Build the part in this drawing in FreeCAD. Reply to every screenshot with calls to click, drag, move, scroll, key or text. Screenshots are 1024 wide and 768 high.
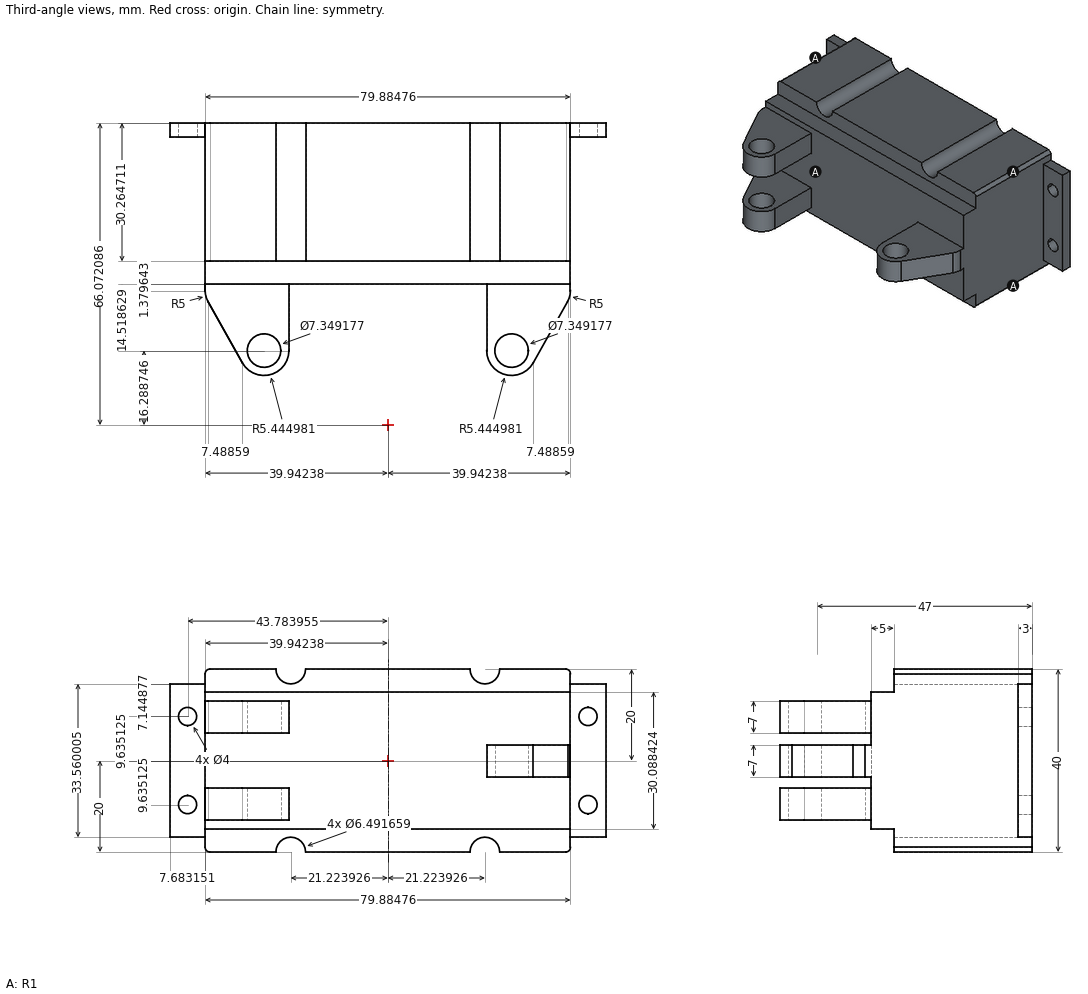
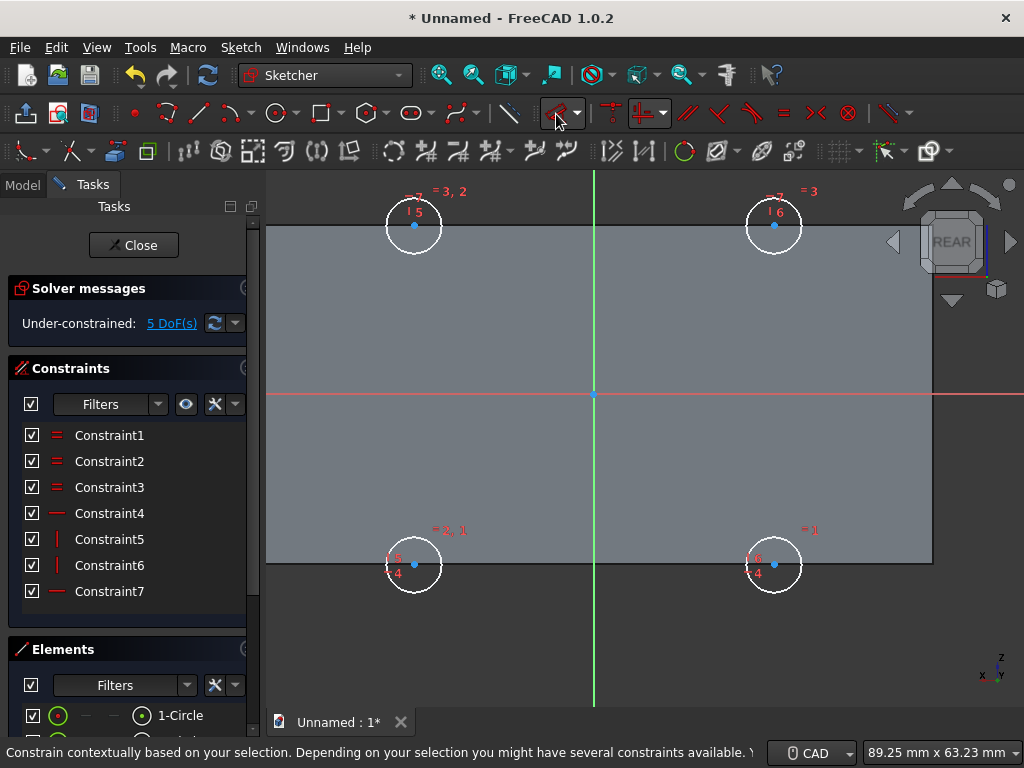
click(793, 545)
click(815, 522)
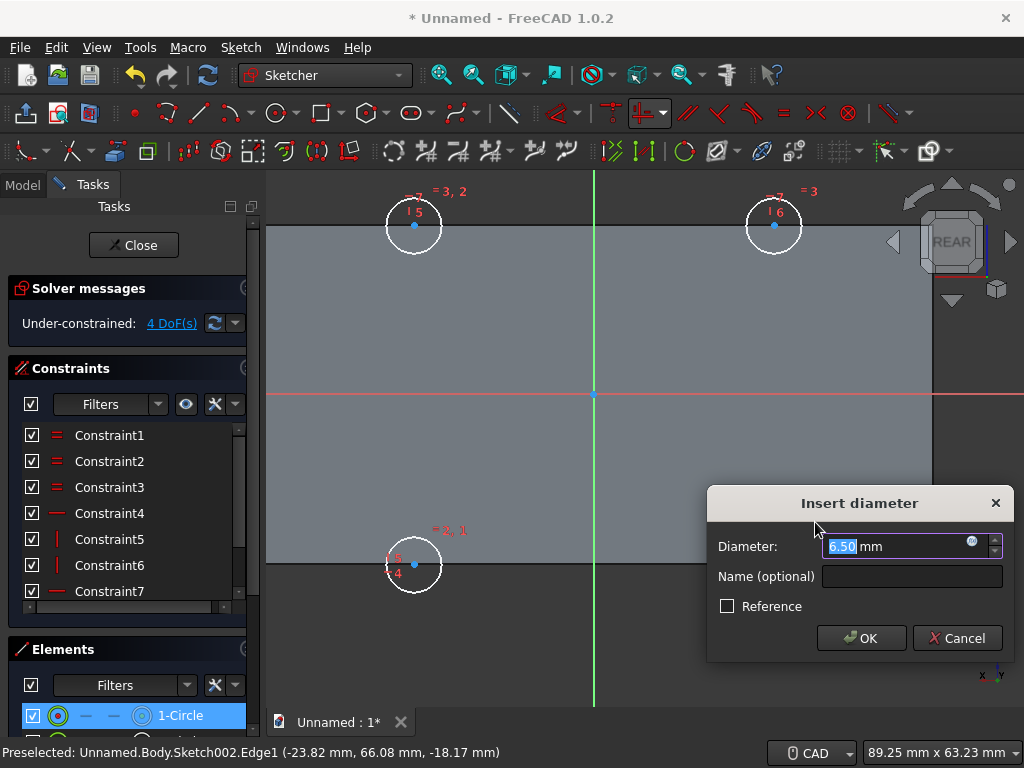
text(6.491659)
key(Return)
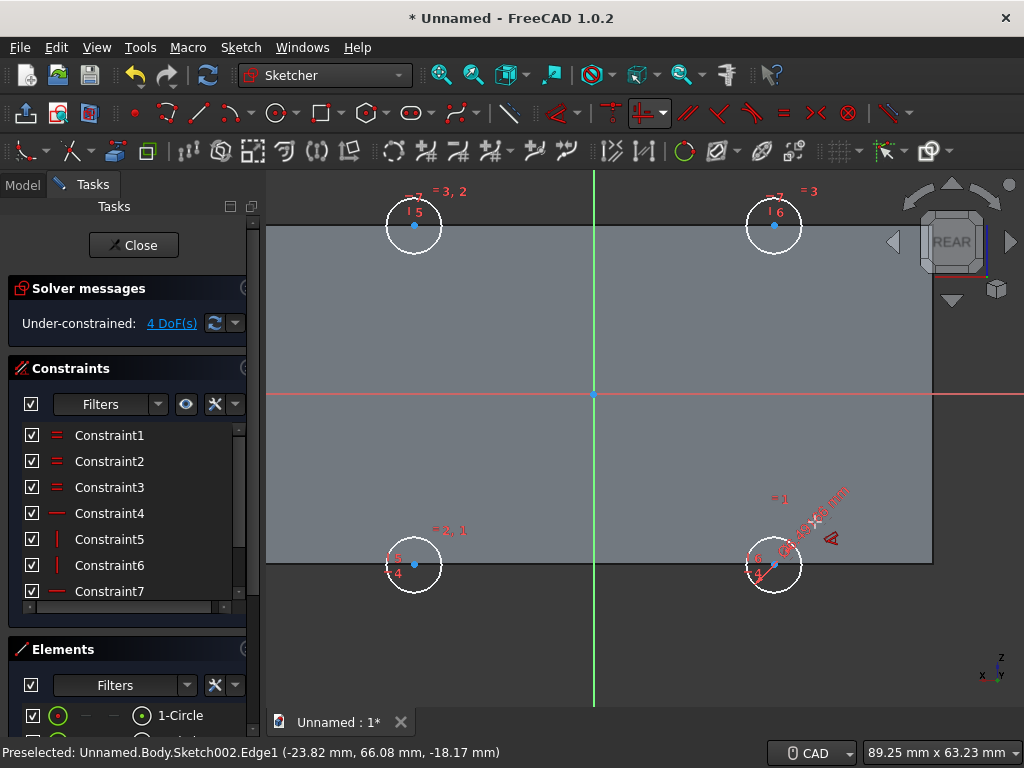
click(774, 565)
click(808, 480)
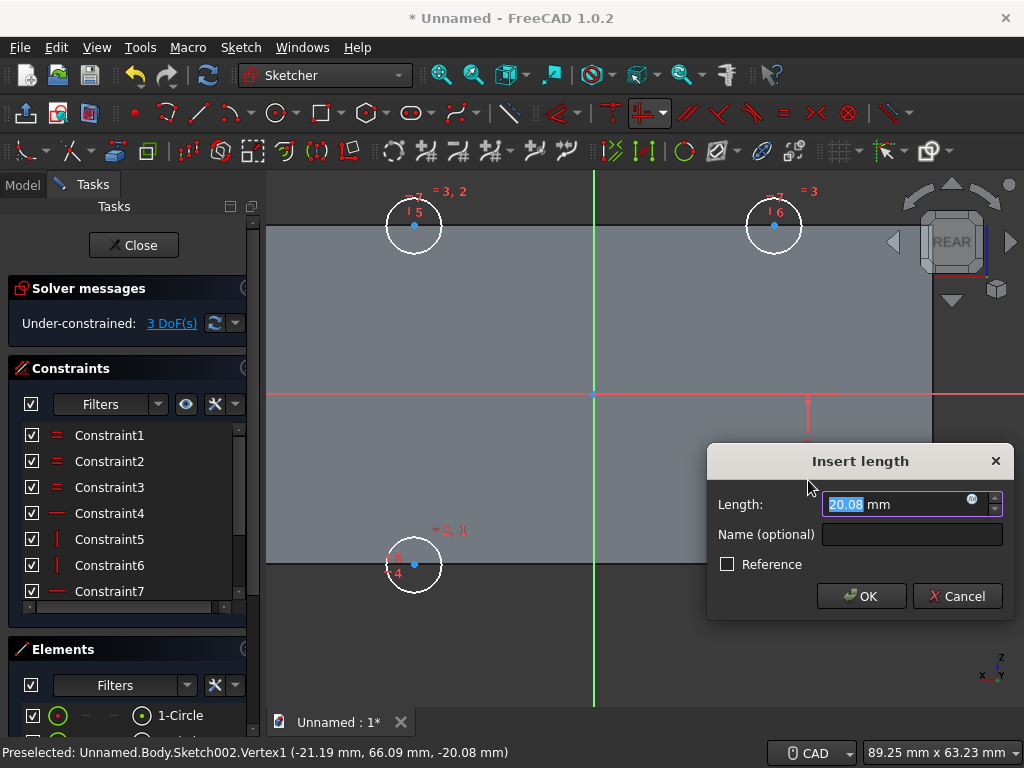
text(20)
key(Return)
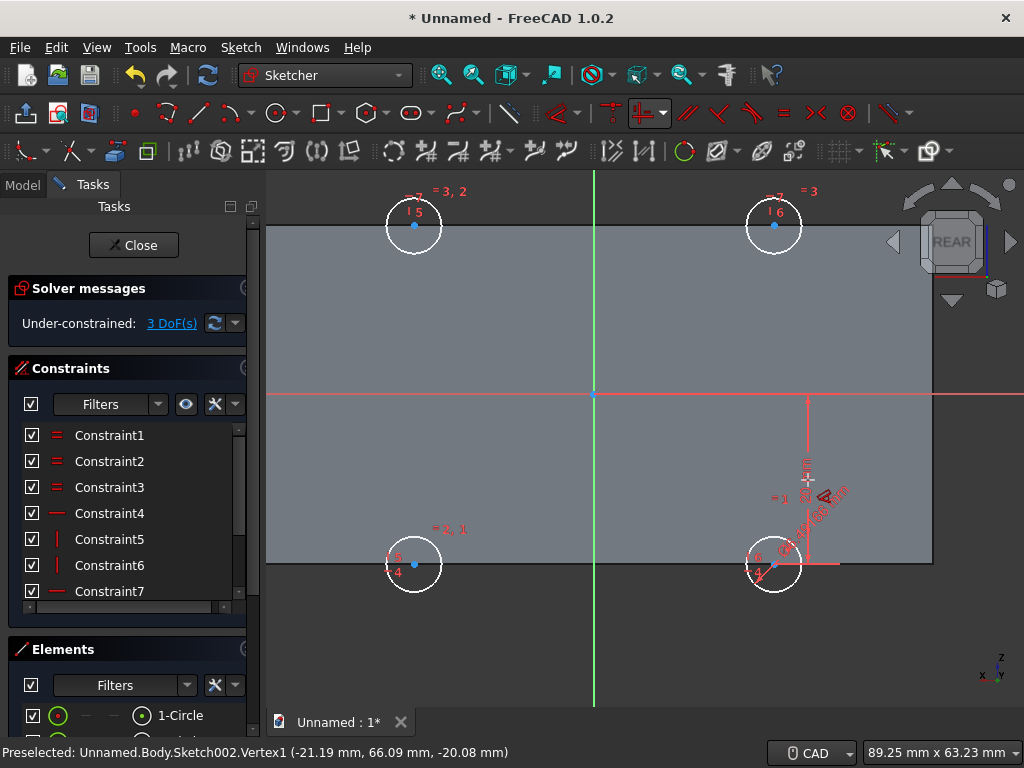
click(414, 226)
click(380, 310)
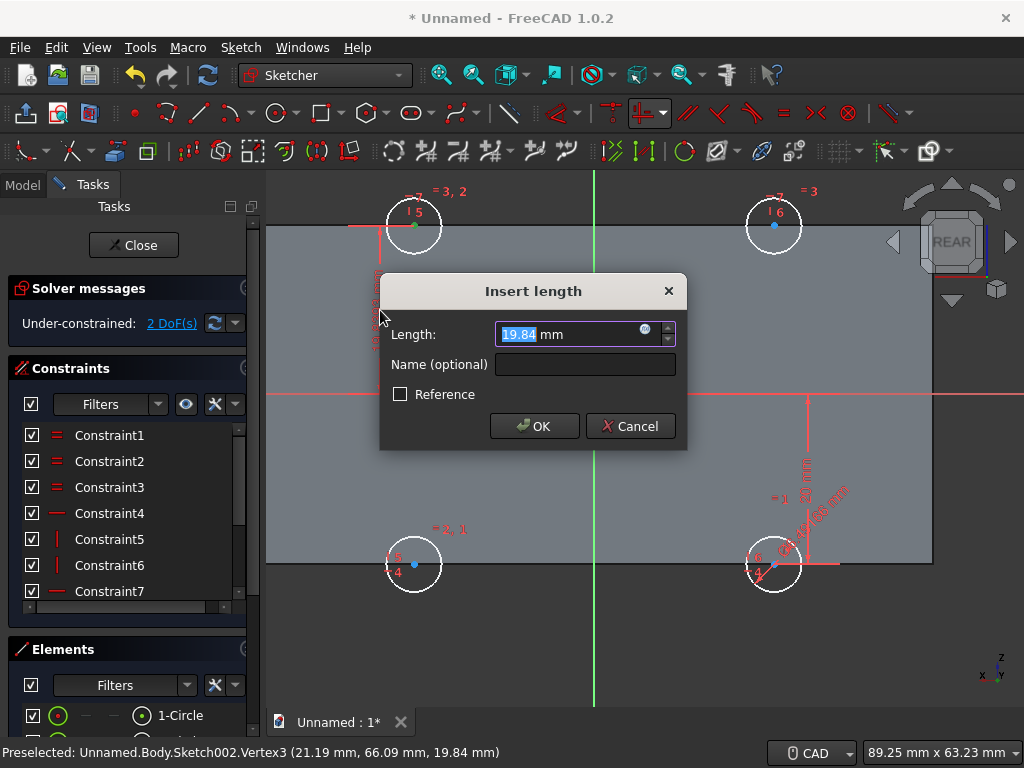
text(20)
key(Return)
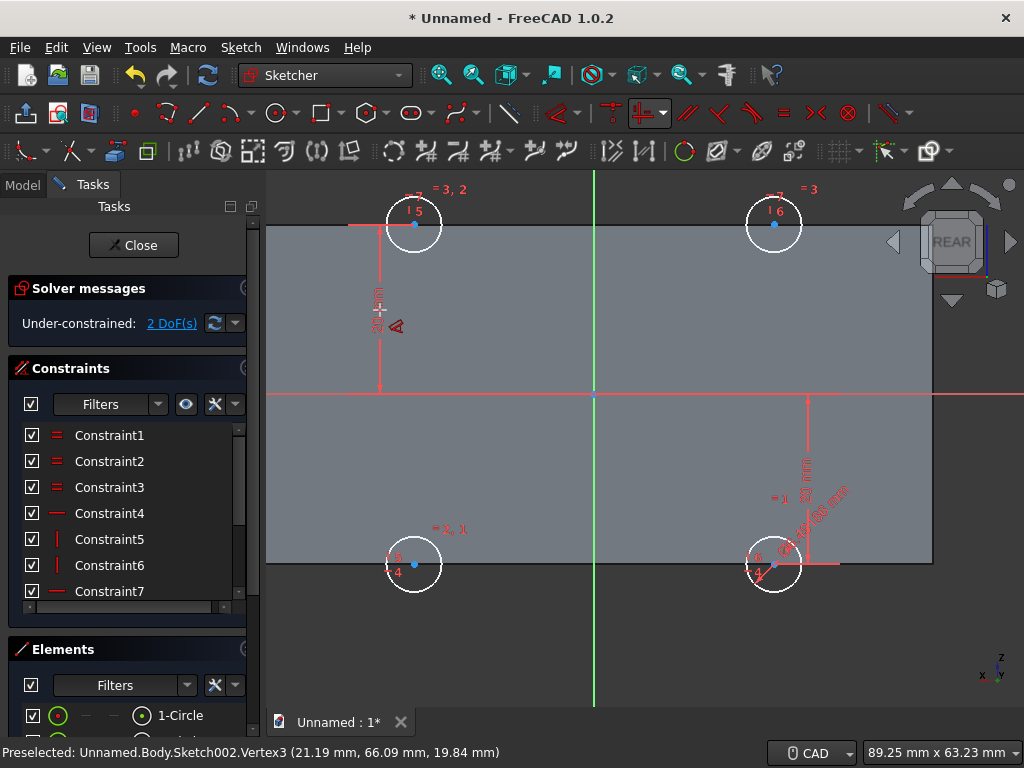
click(774, 564)
click(684, 598)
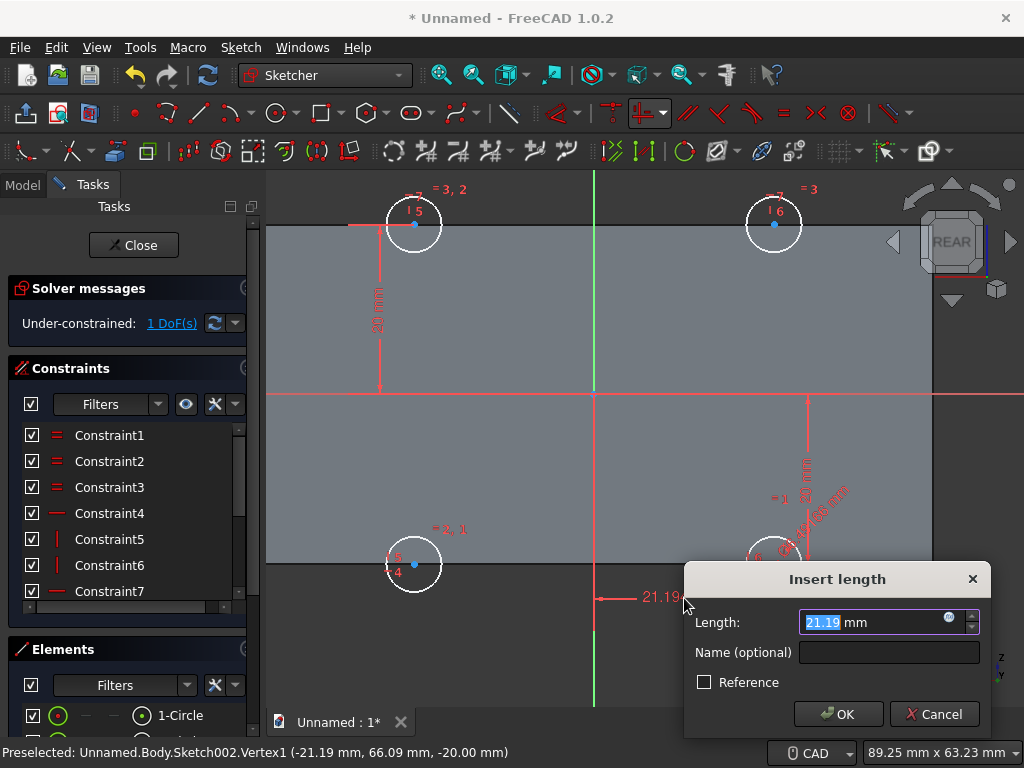
text(21.223926)
key(Return)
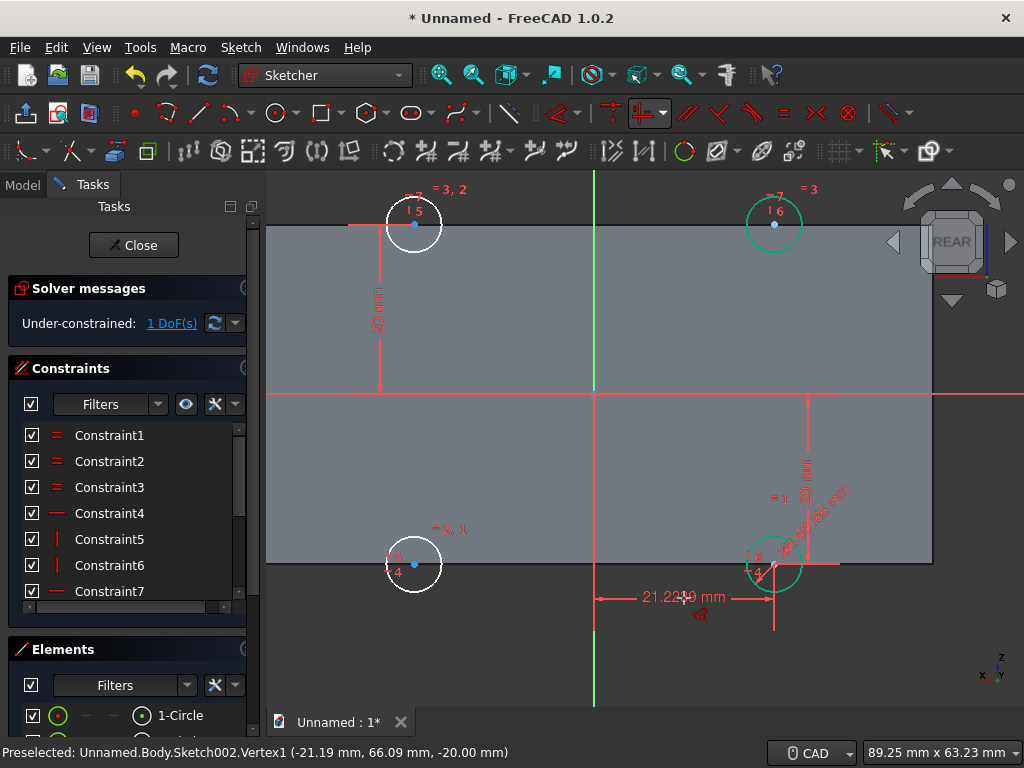
click(414, 564)
click(504, 598)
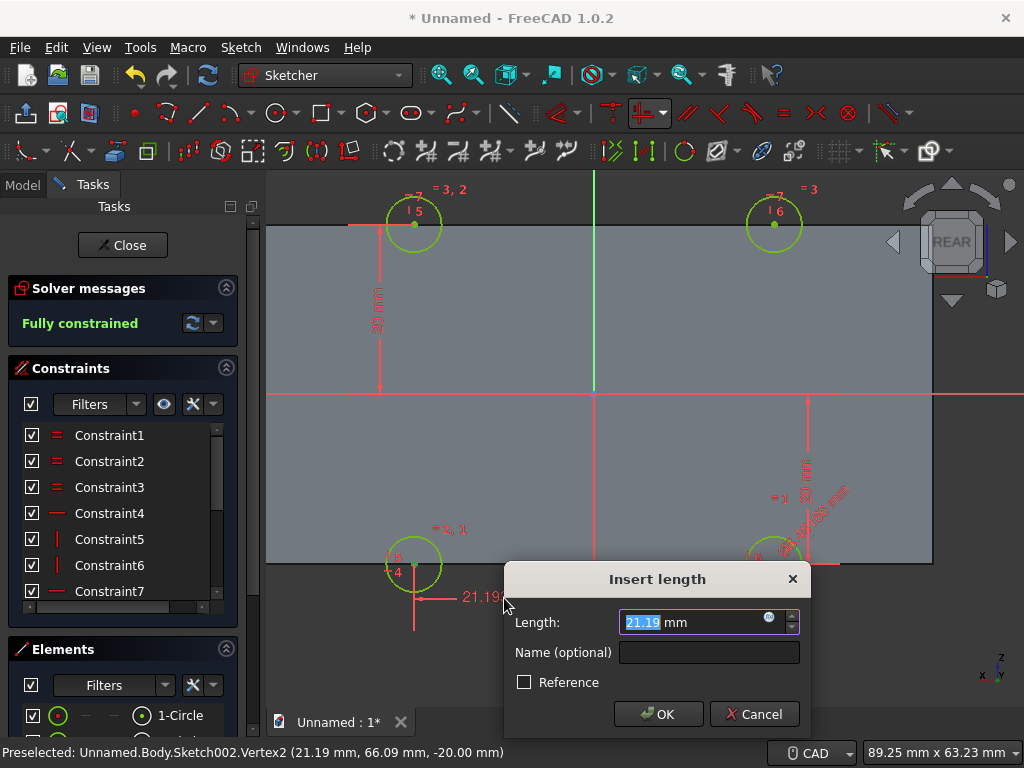
text(21.223926)
key(Return)
key(Escape)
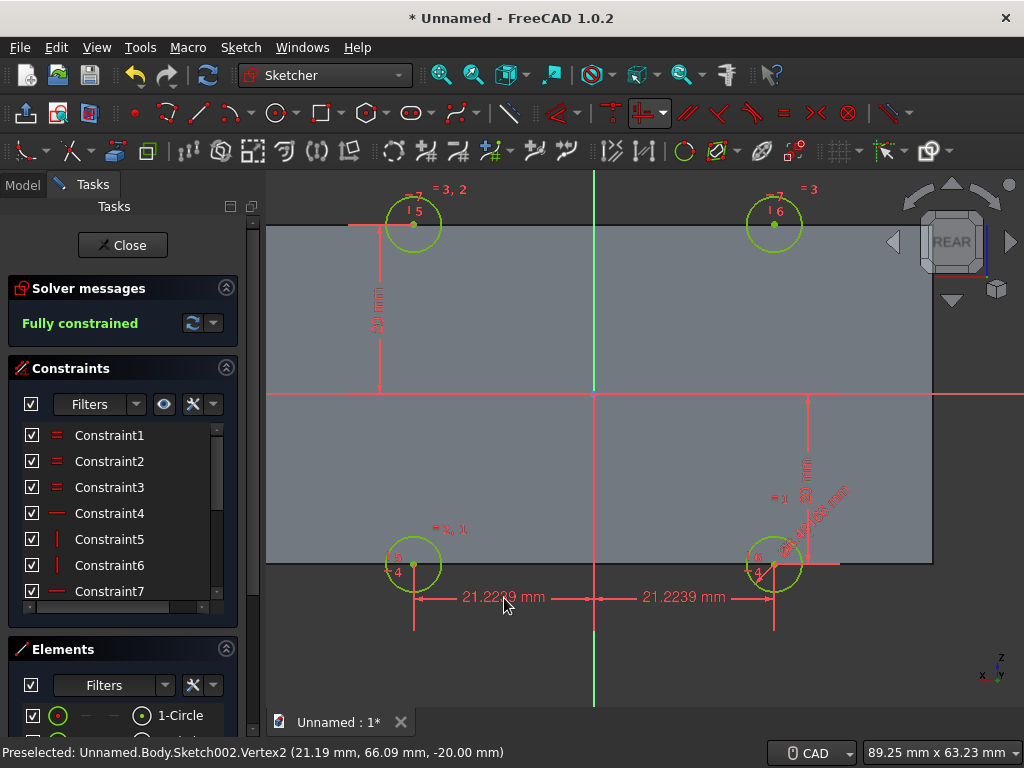
click(123, 245)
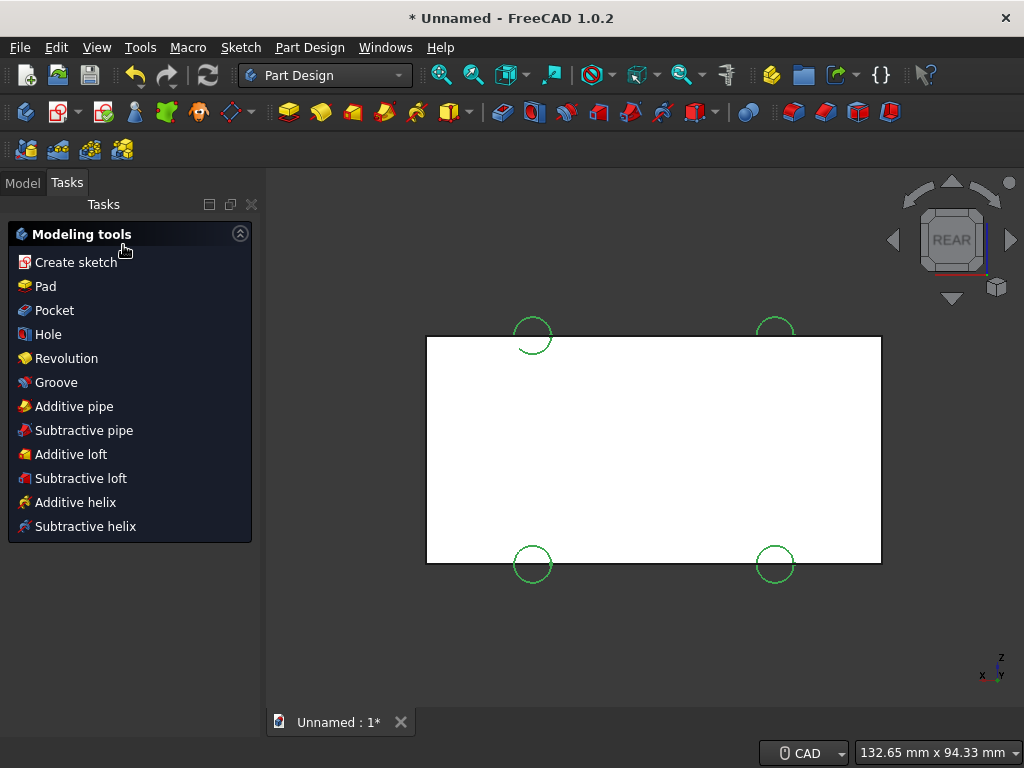
click(504, 112)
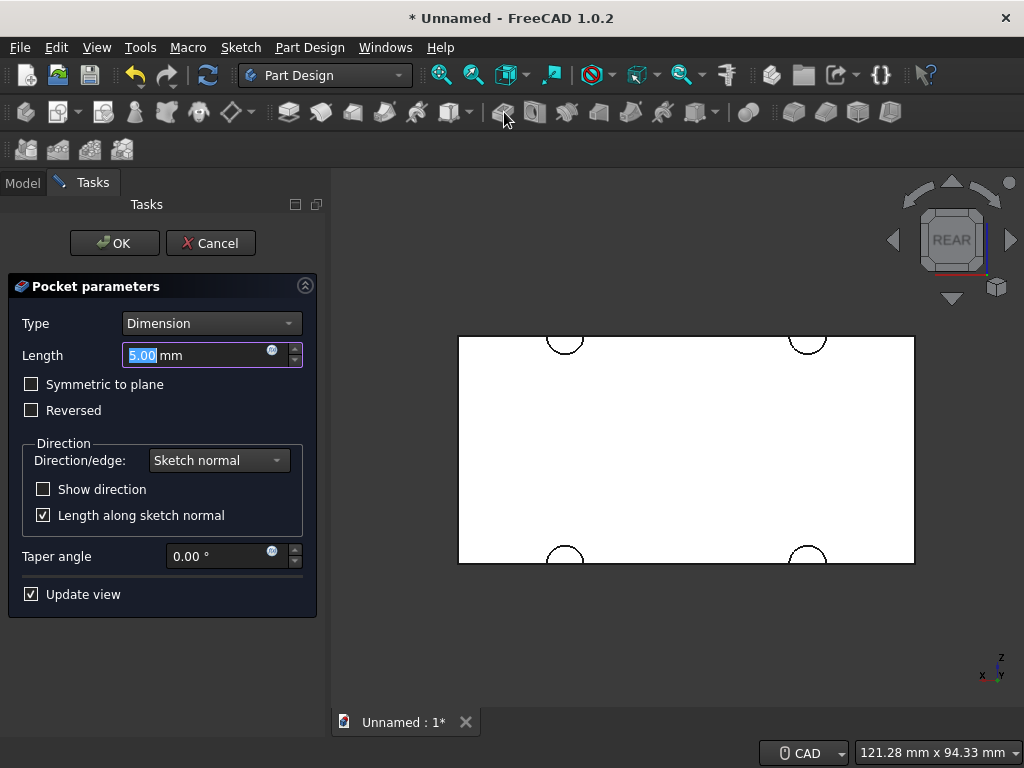
text(47)
key(Tab)